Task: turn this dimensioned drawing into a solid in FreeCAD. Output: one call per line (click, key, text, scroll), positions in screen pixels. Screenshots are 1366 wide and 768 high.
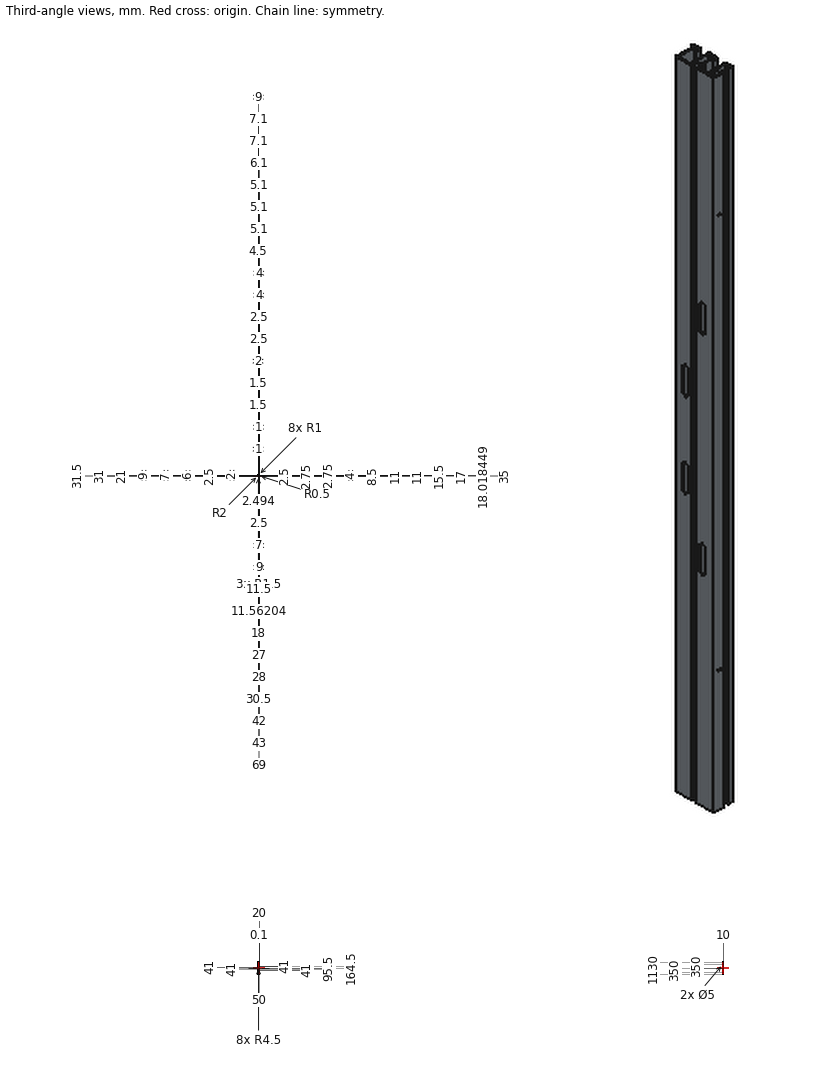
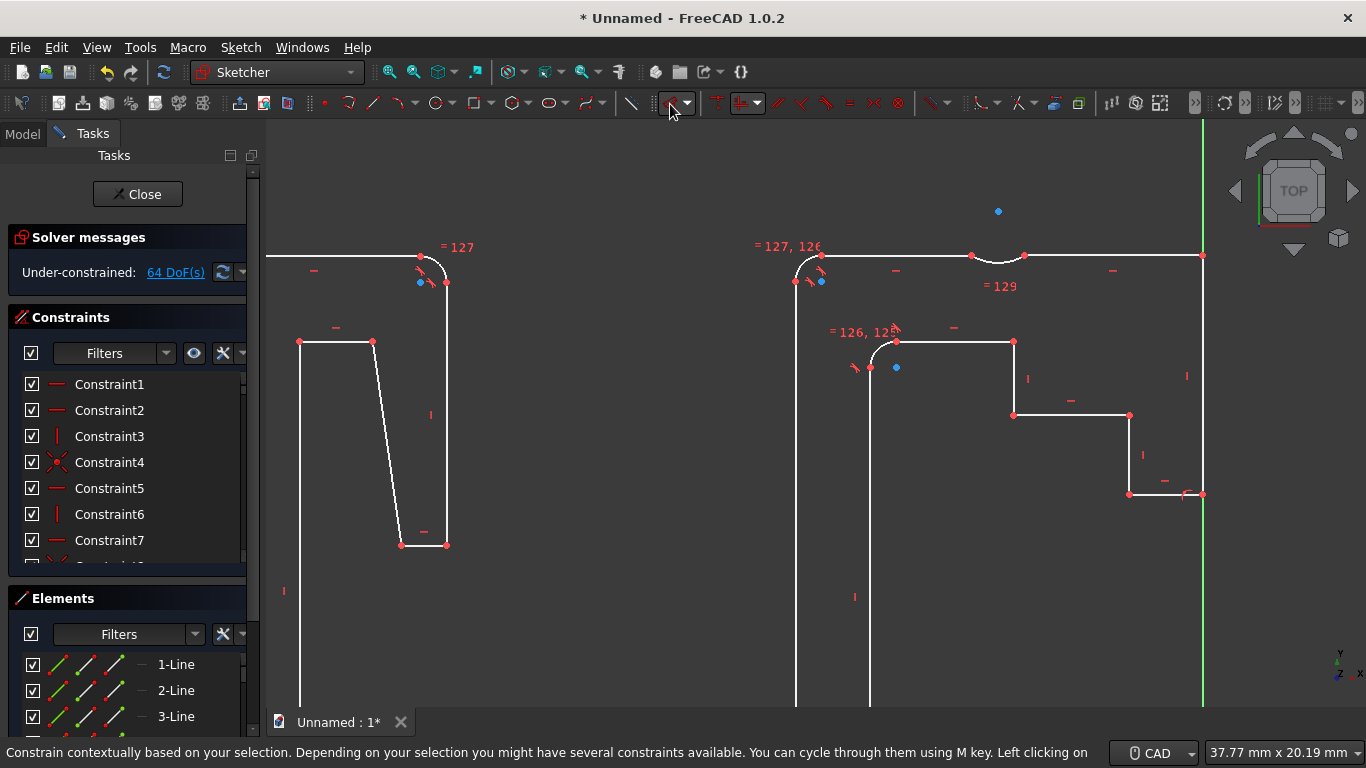
scroll(991, 262, down, 6)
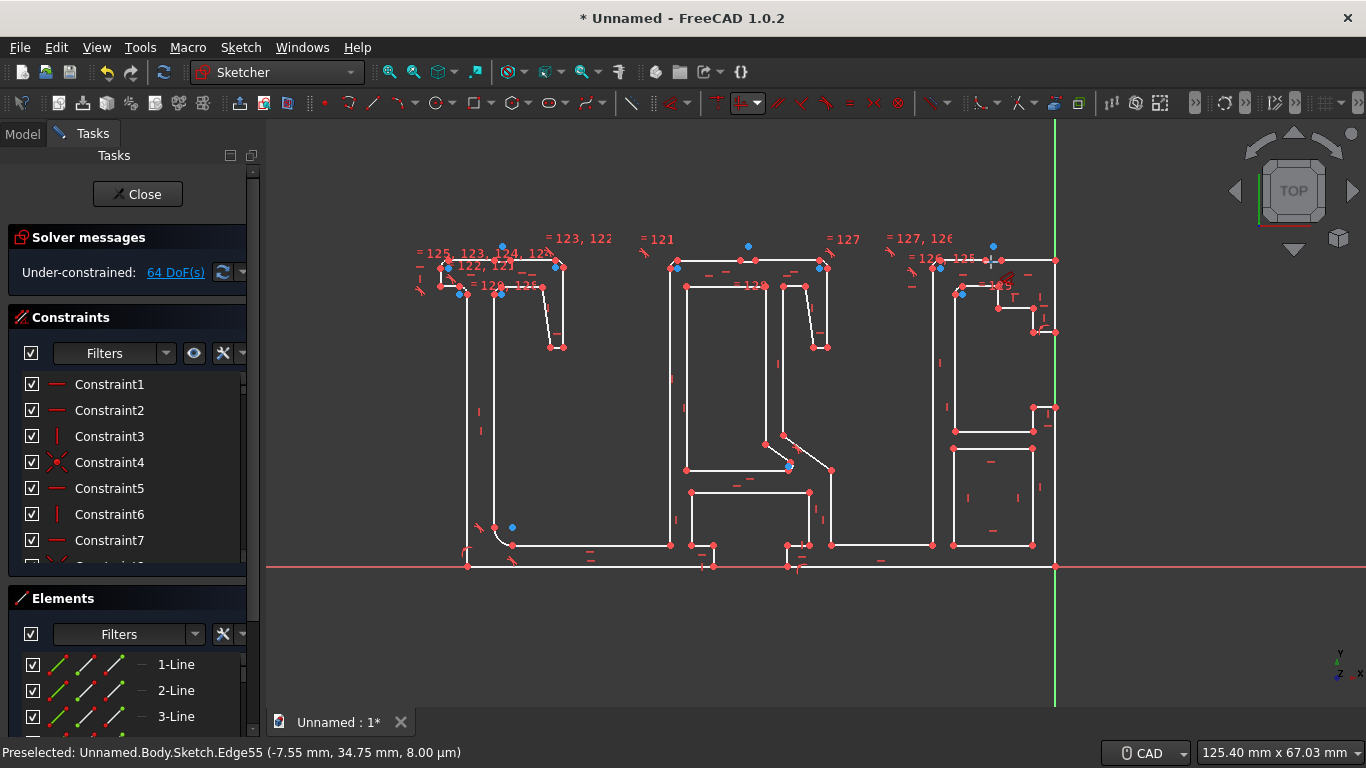
scroll(745, 262, up, 6)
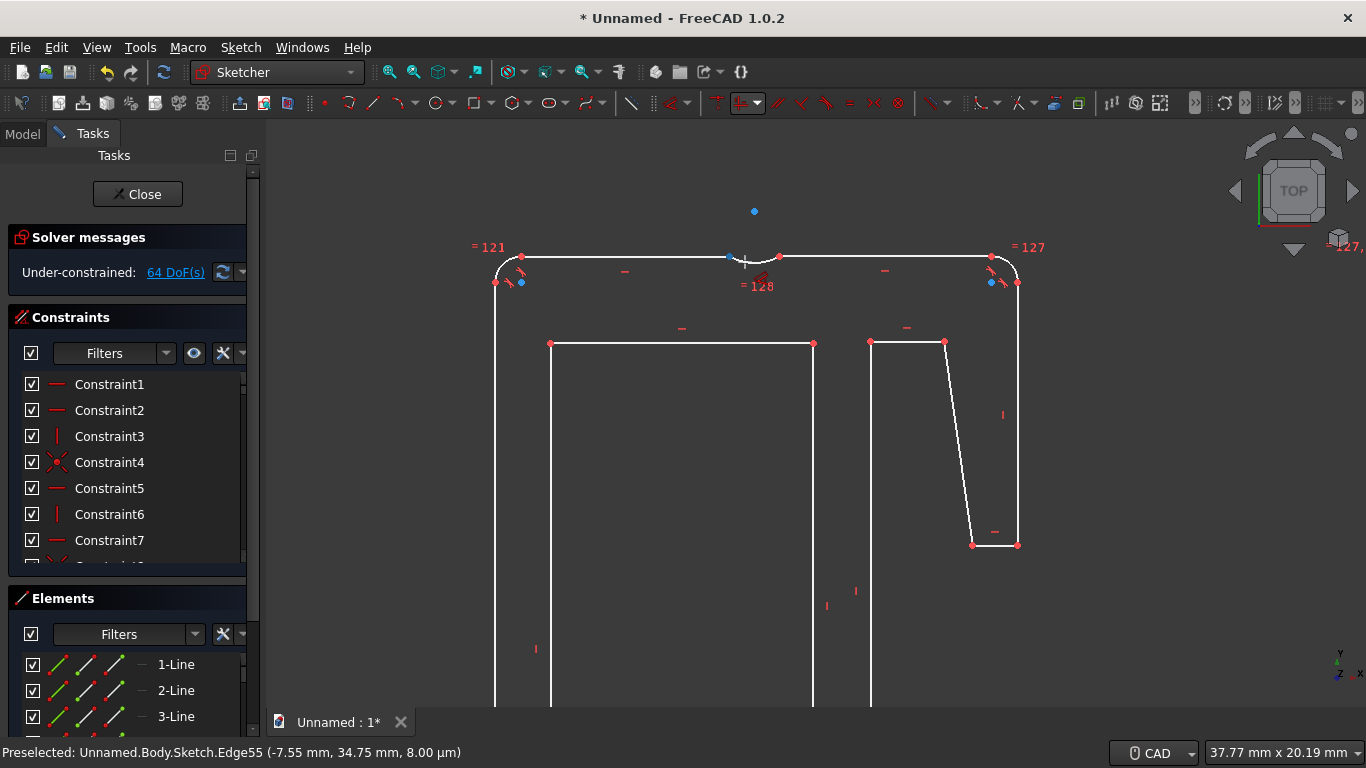
click(745, 262)
click(739, 293)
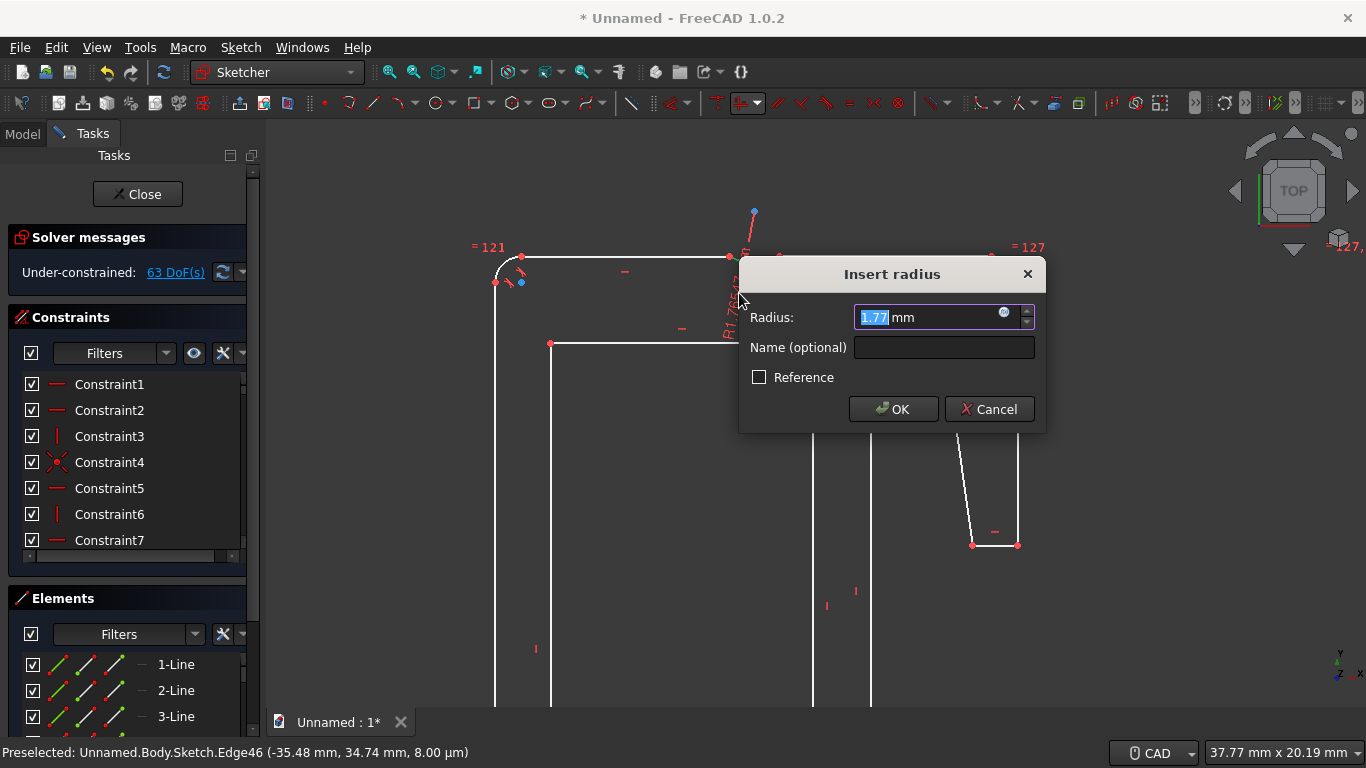
text(1.5)
key(Return)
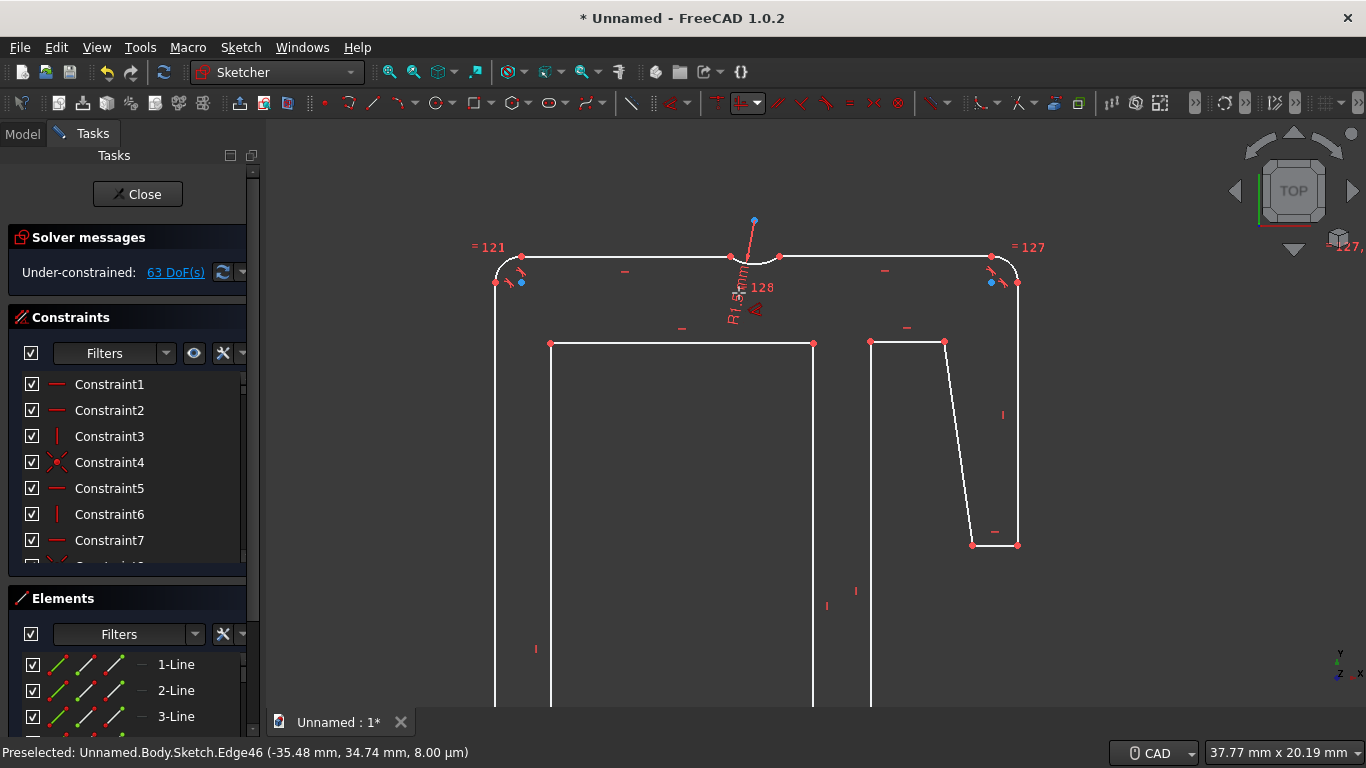
scroll(509, 260, up, 2)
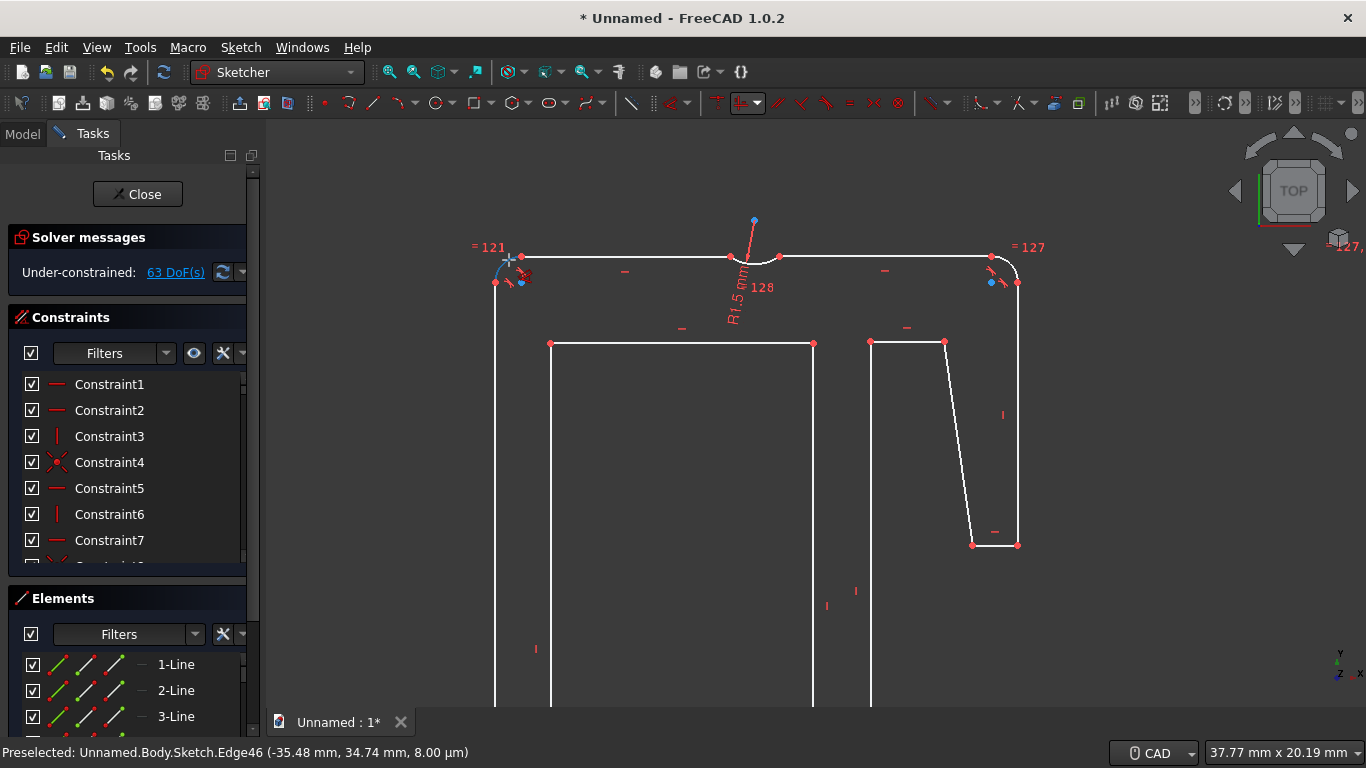
click(510, 259)
click(496, 230)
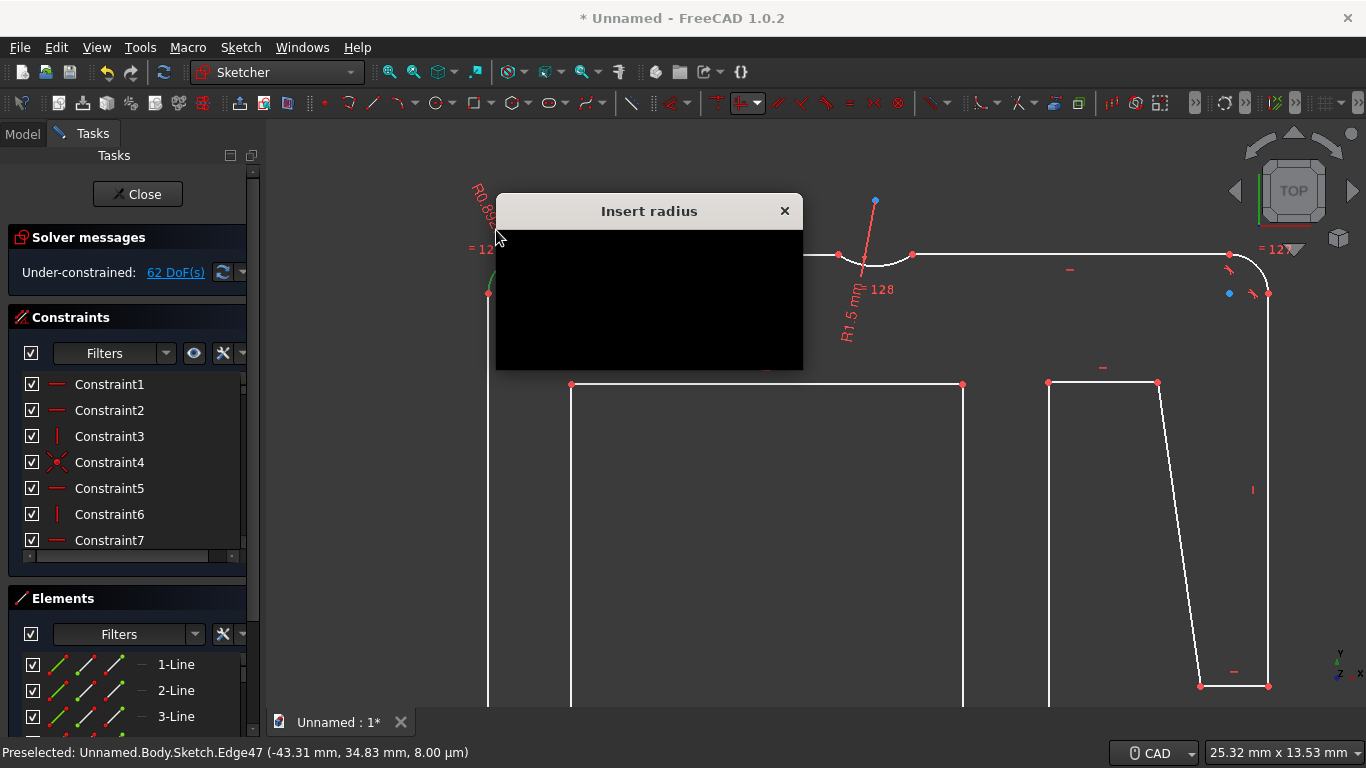
text(1)
key(Return)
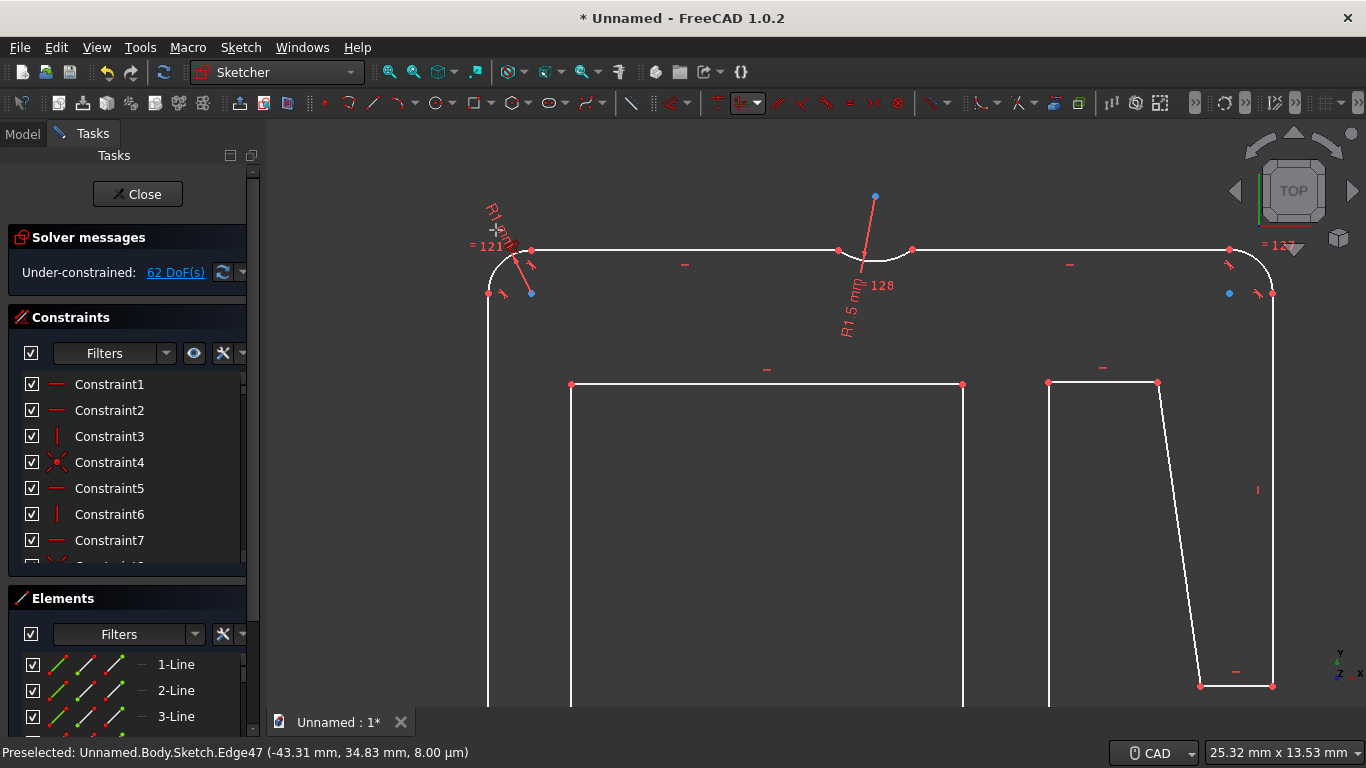
scroll(715, 262, down, 8)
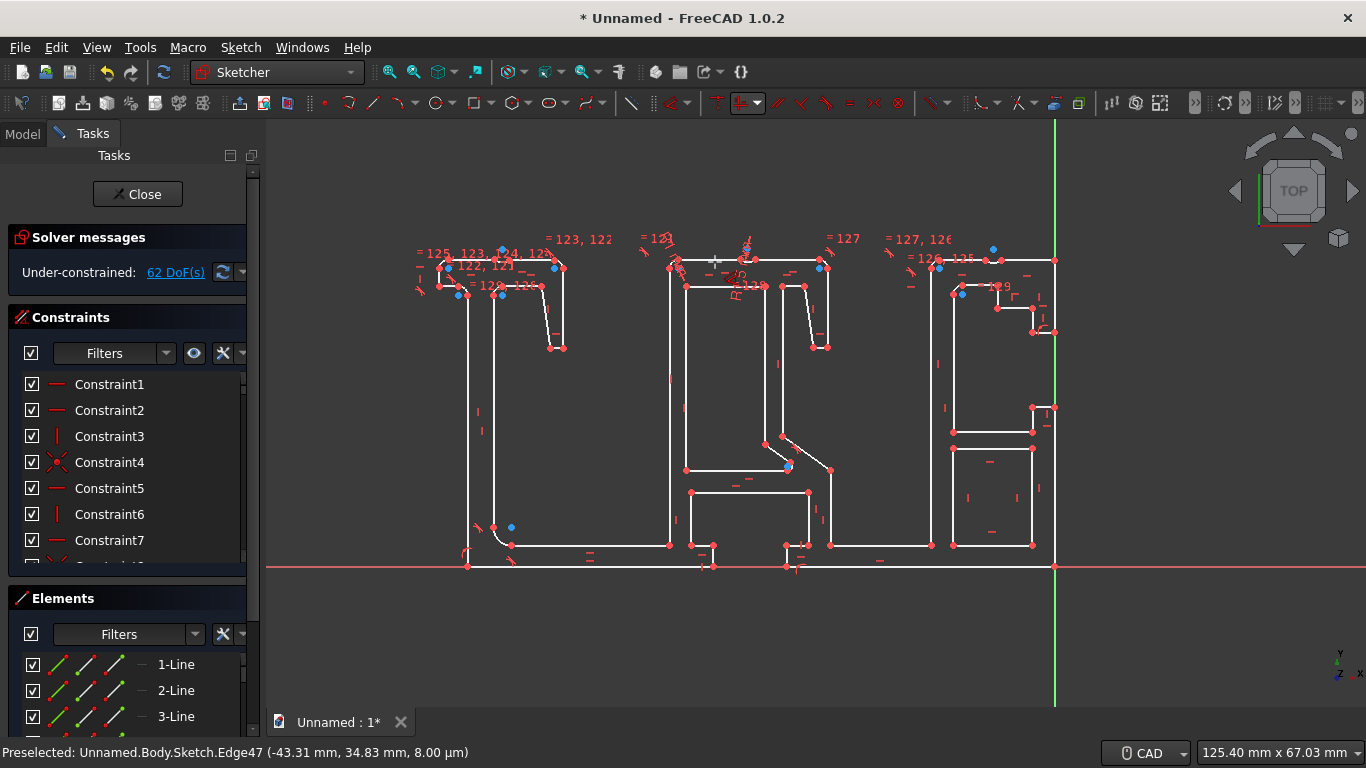
scroll(496, 536, up, 5)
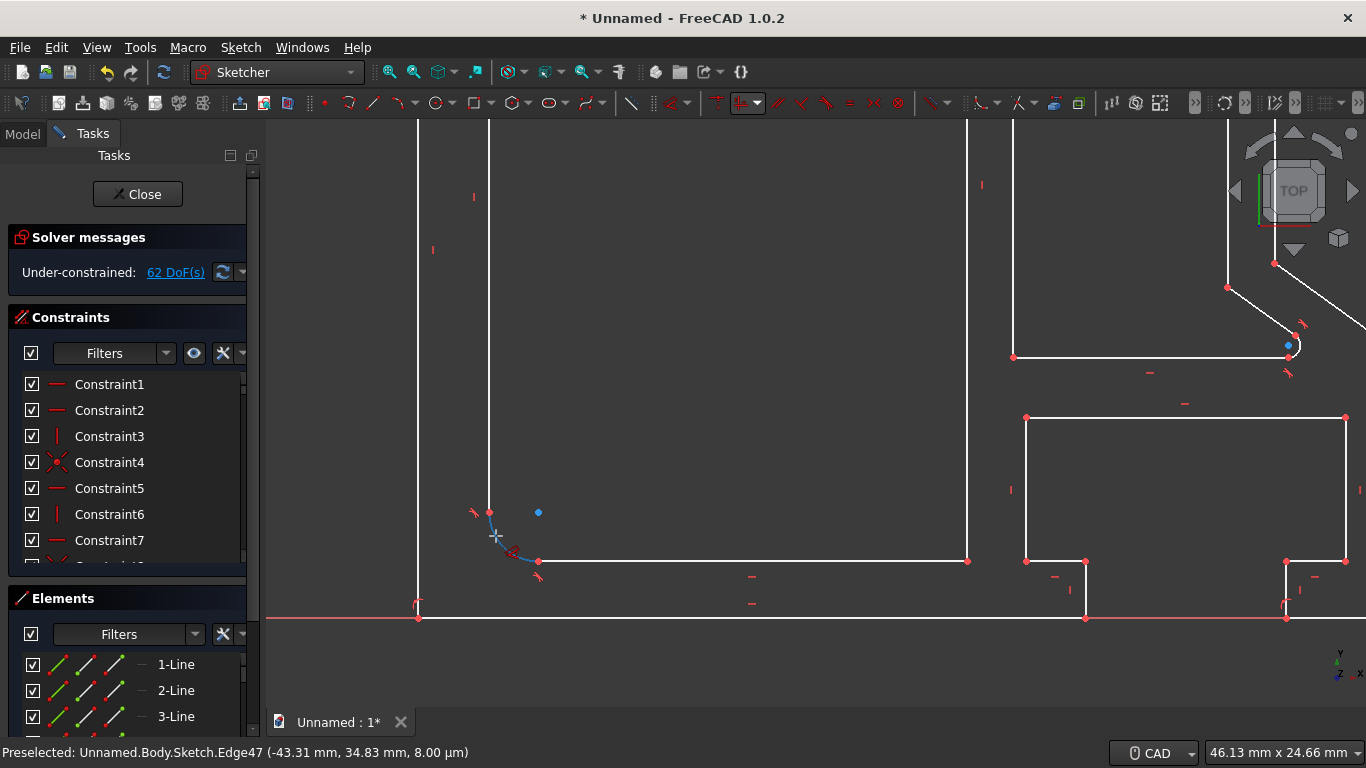
click(495, 535)
click(467, 550)